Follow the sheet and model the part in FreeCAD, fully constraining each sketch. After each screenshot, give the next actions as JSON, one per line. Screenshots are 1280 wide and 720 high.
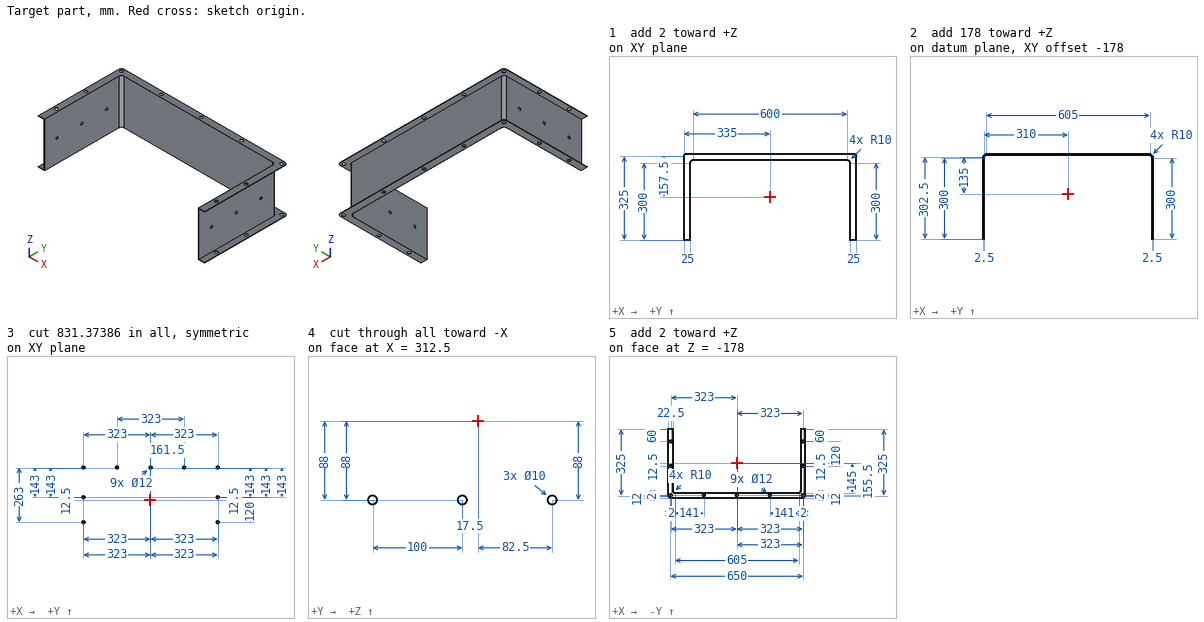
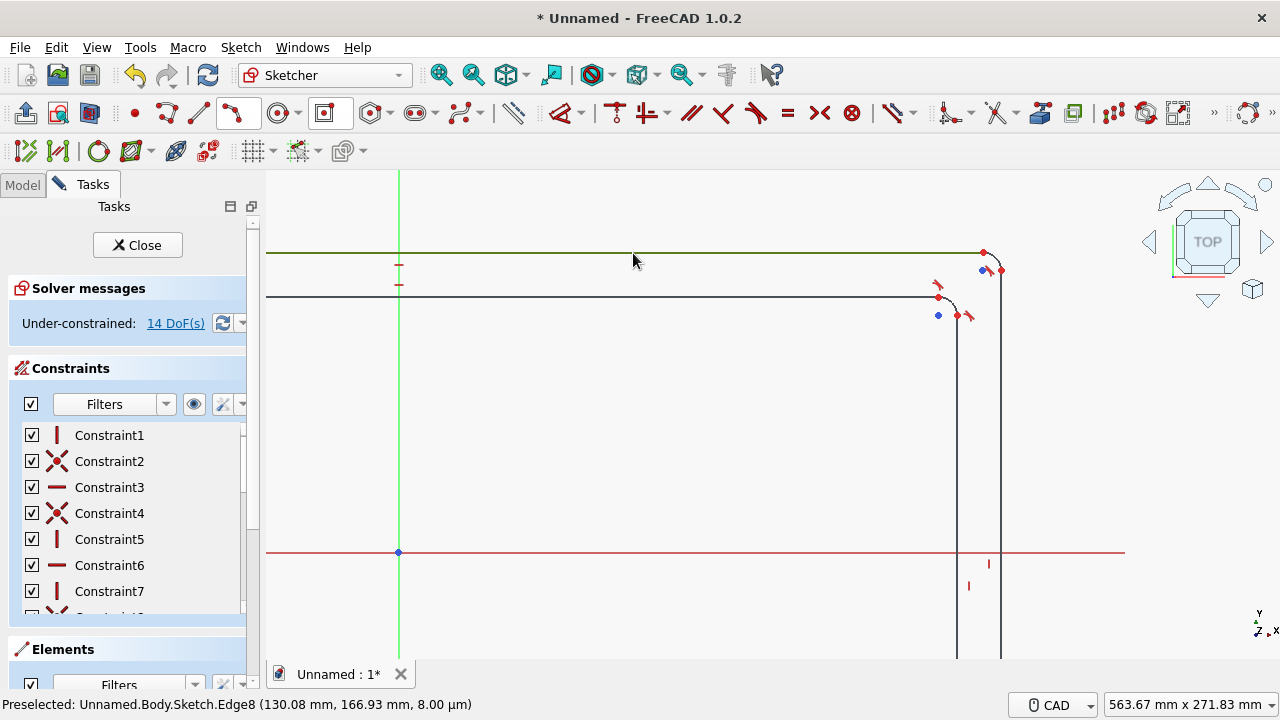
{"action": "left_click", "coordinate": [996, 258]}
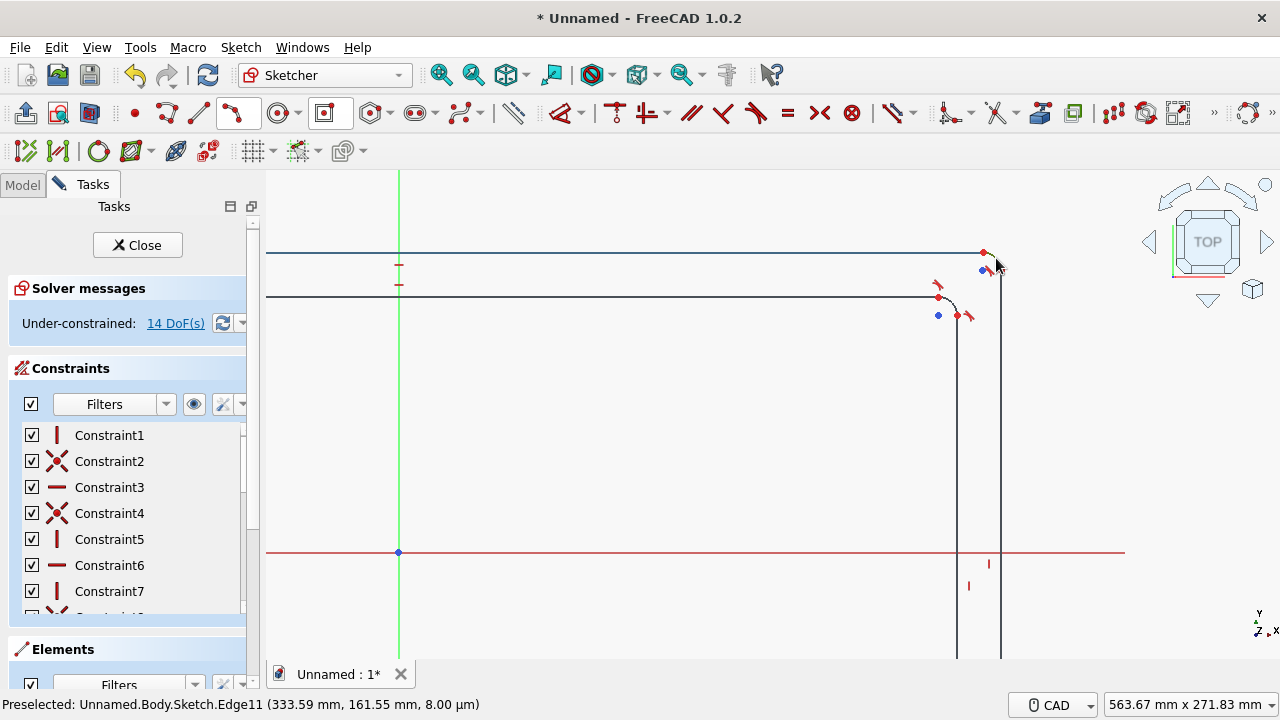
{"action": "key", "text": "t"}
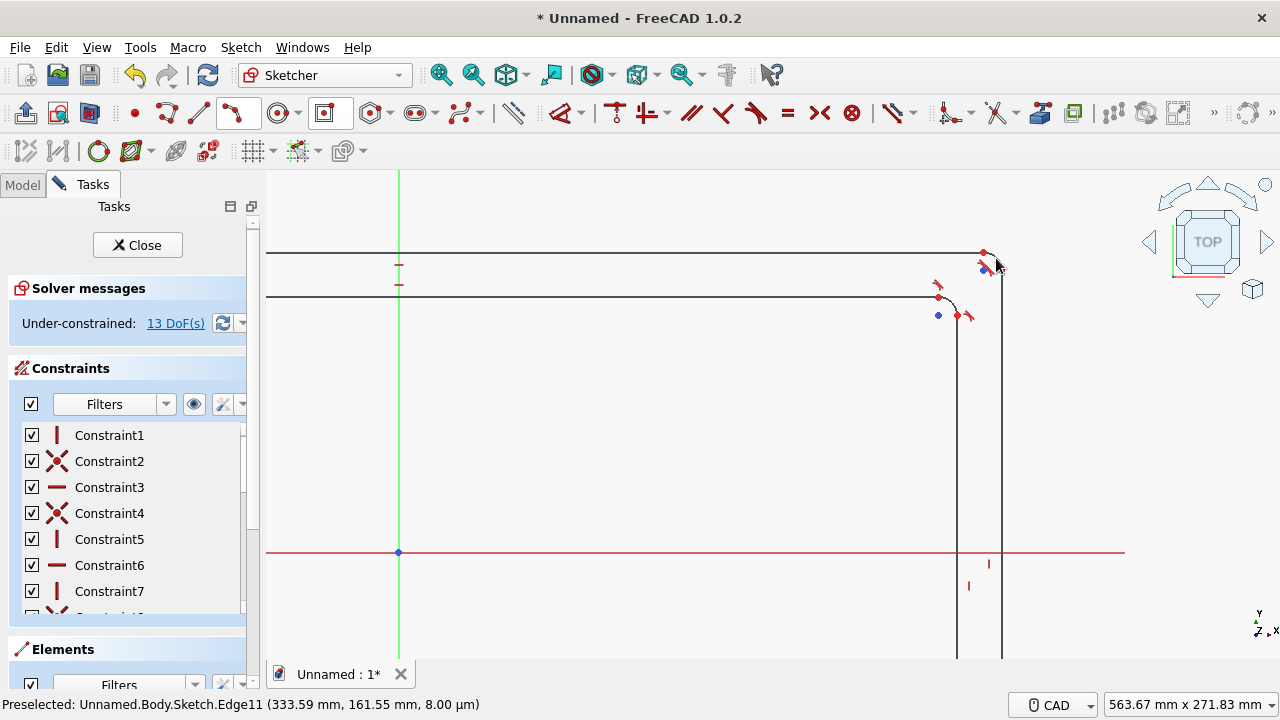
{"action": "left_click", "coordinate": [633, 253]}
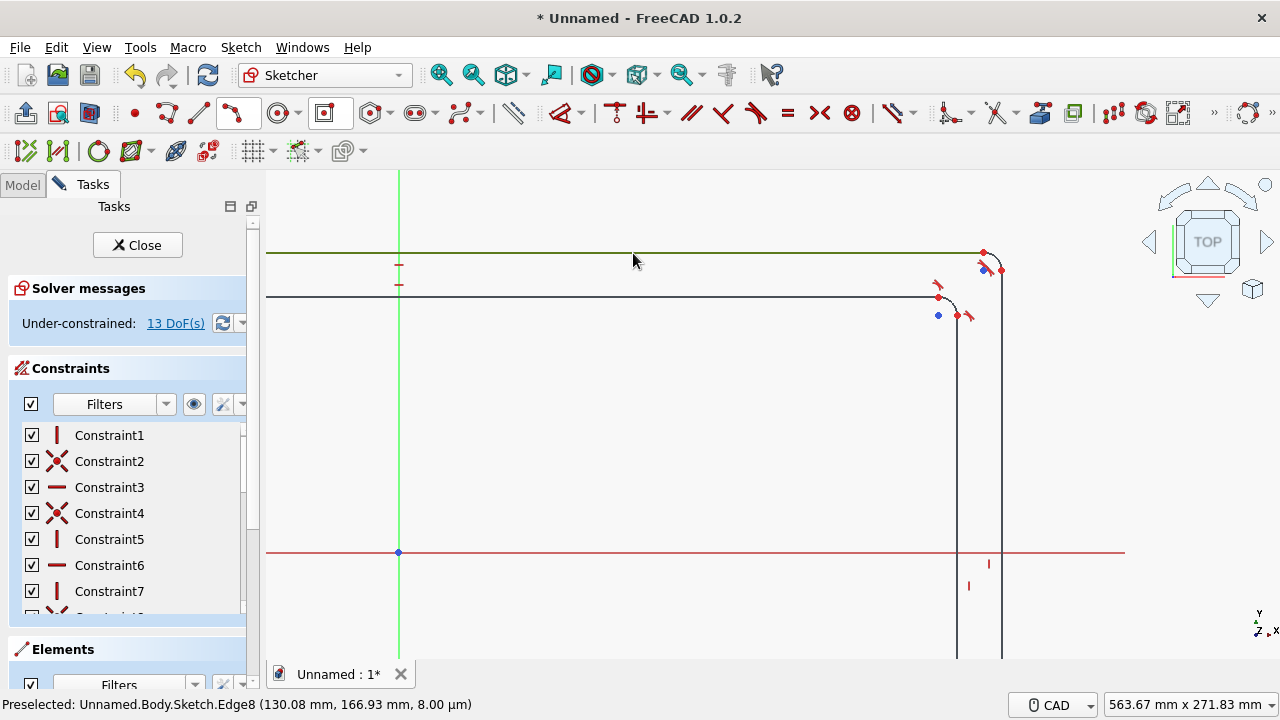
{"action": "scroll", "coordinate": [954, 302], "scroll_direction": "down", "scroll_amount": 4}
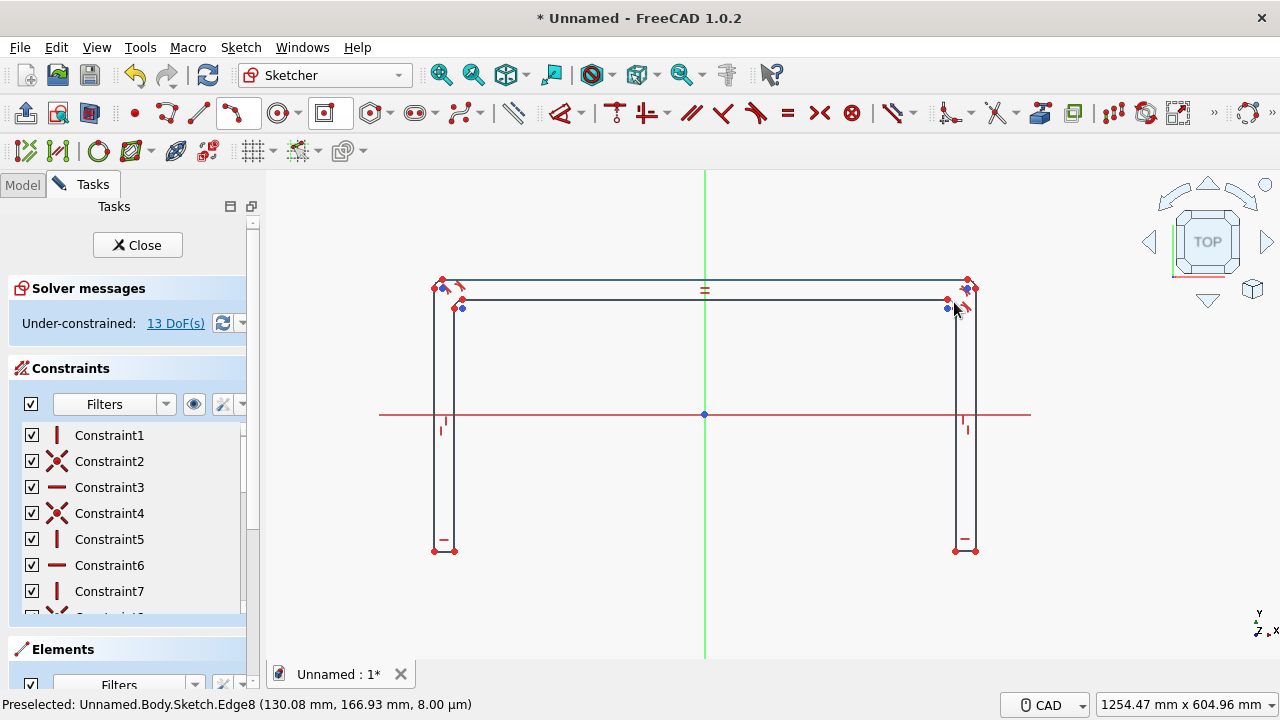
{"action": "scroll", "coordinate": [436, 282], "scroll_direction": "up", "scroll_amount": 4}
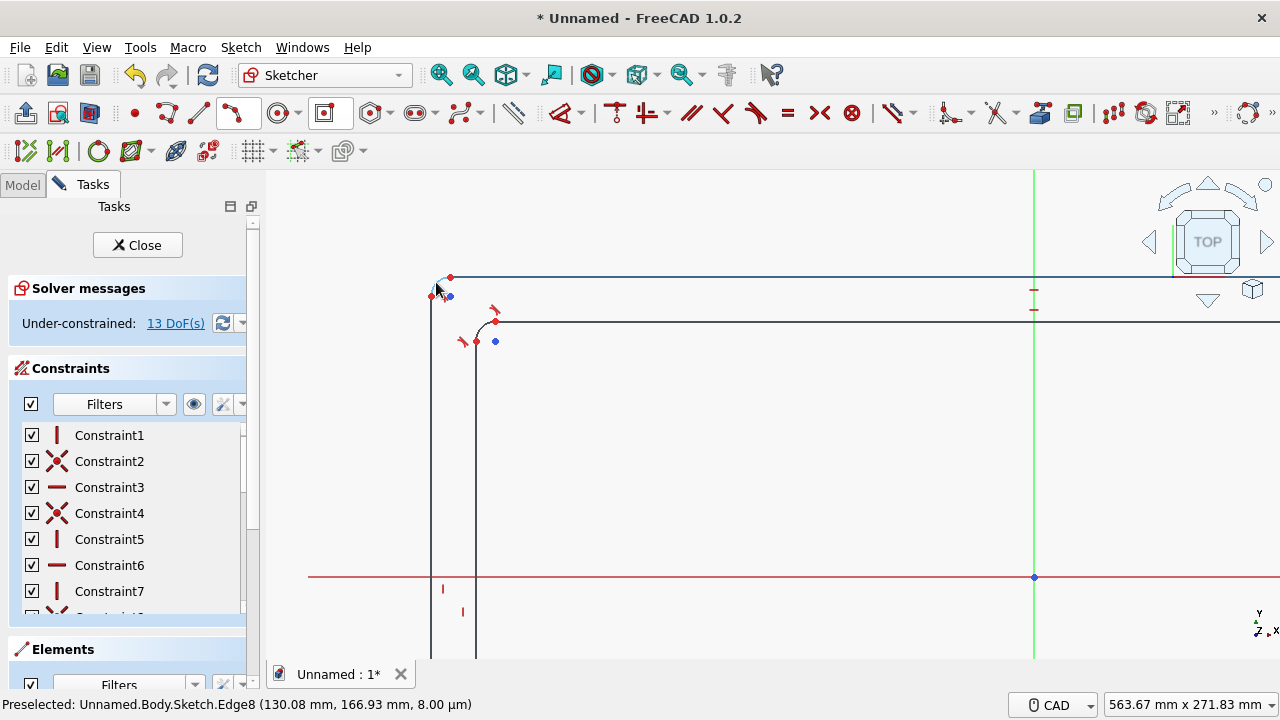
{"action": "left_click", "coordinate": [437, 283]}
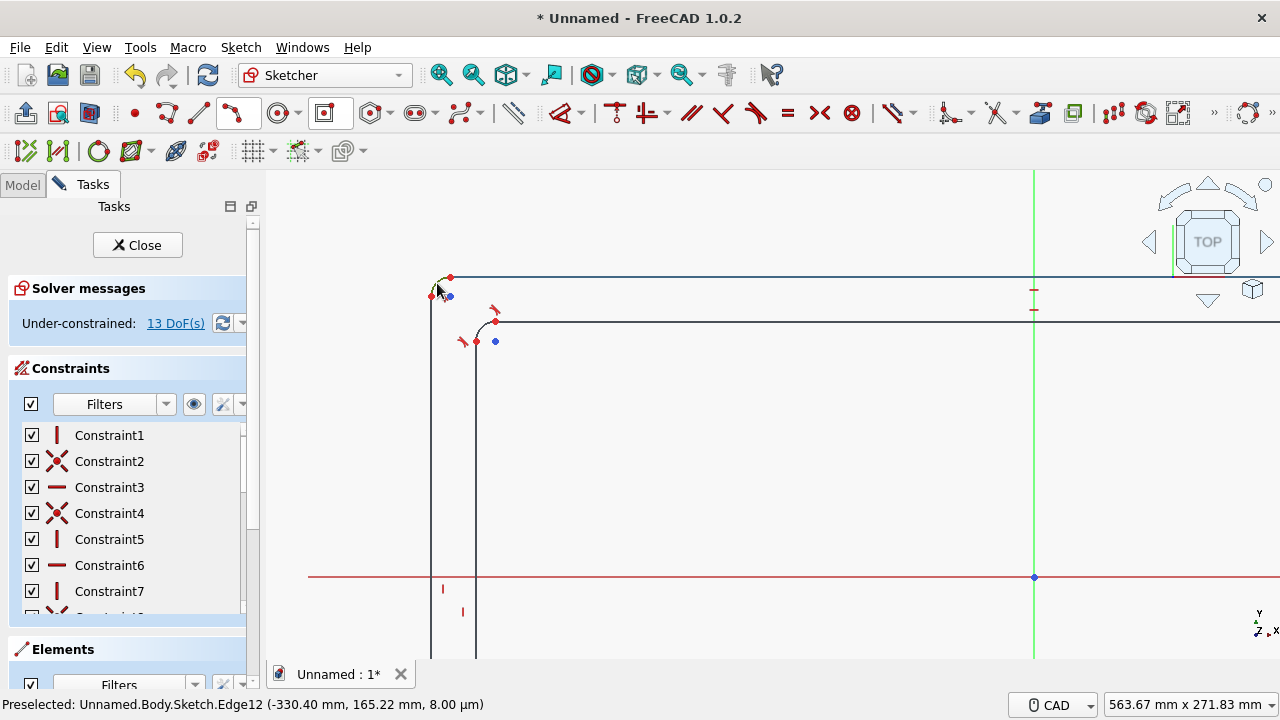
{"action": "left_click", "coordinate": [756, 114]}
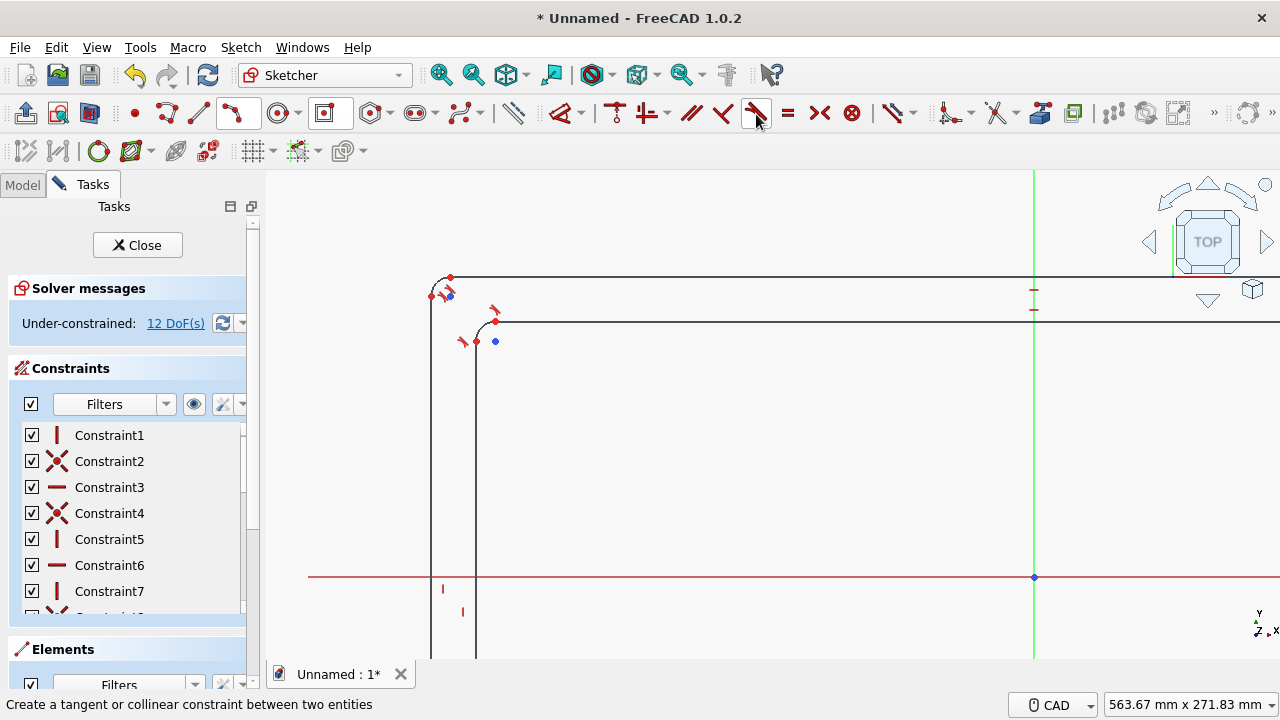
{"action": "scroll", "coordinate": [487, 324], "scroll_direction": "up", "scroll_amount": 3}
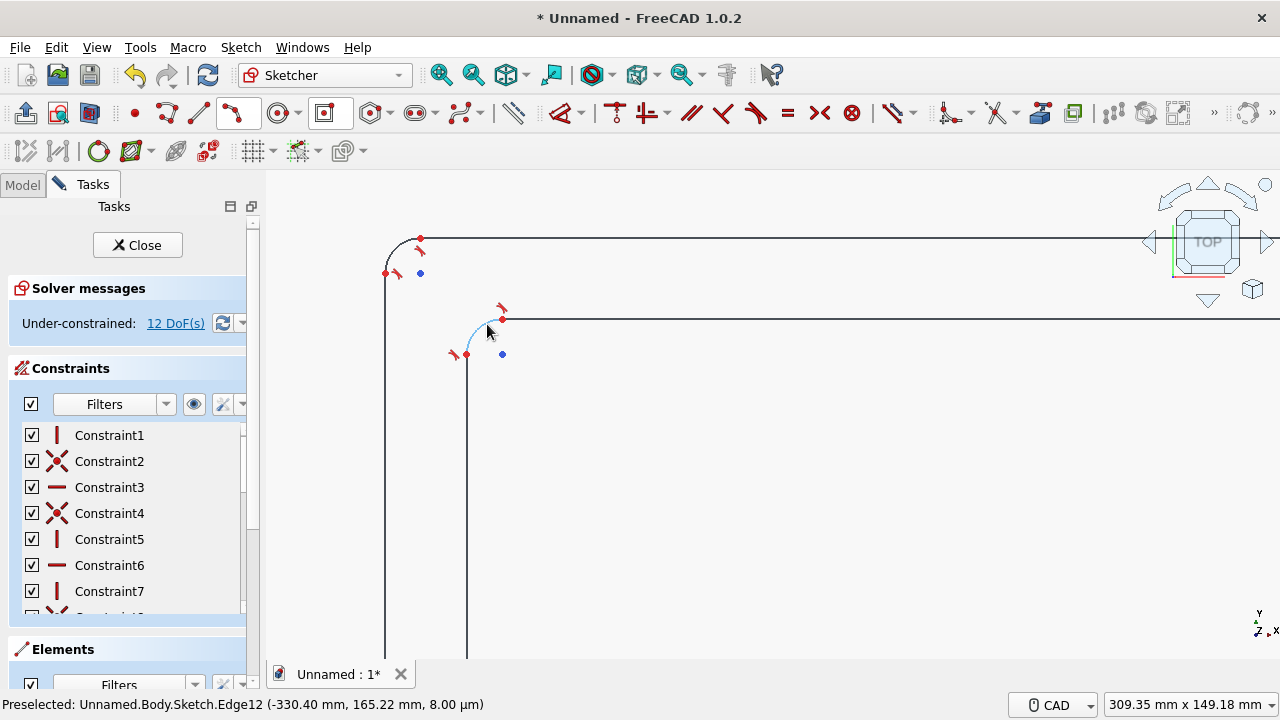
{"action": "left_click", "coordinate": [486, 323]}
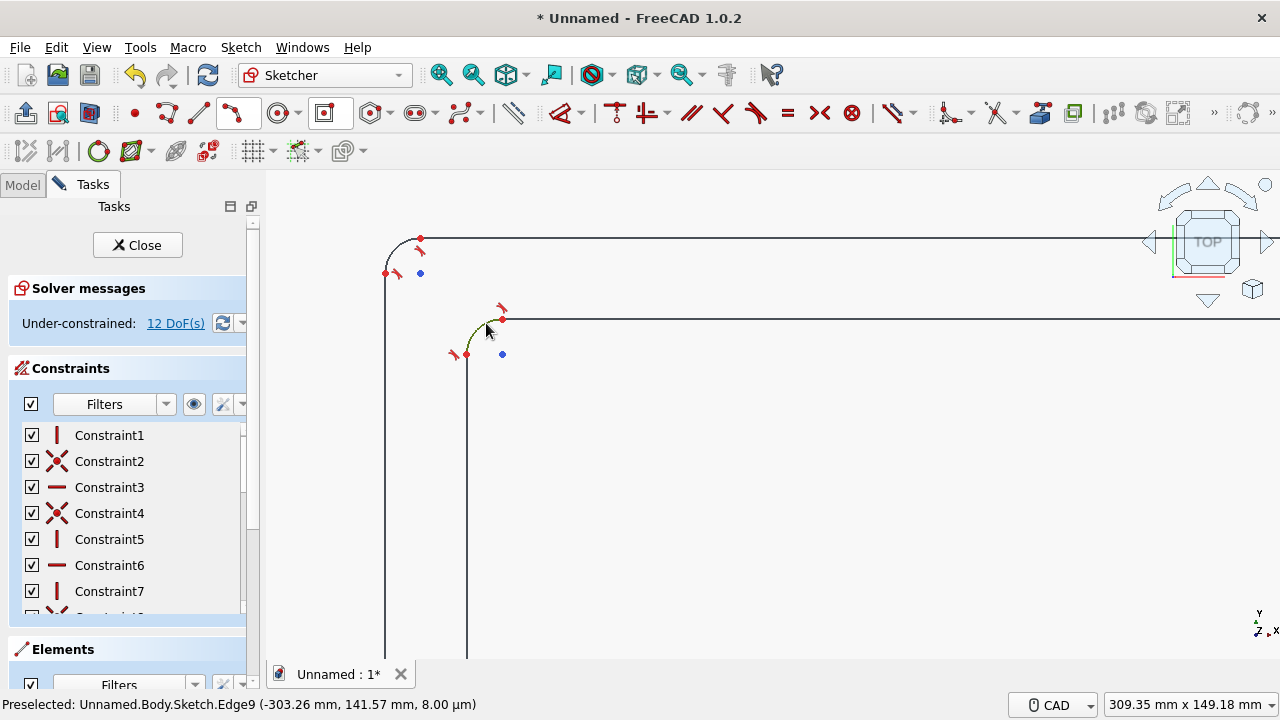
{"action": "scroll", "coordinate": [449, 293], "scroll_direction": "down", "scroll_amount": 7}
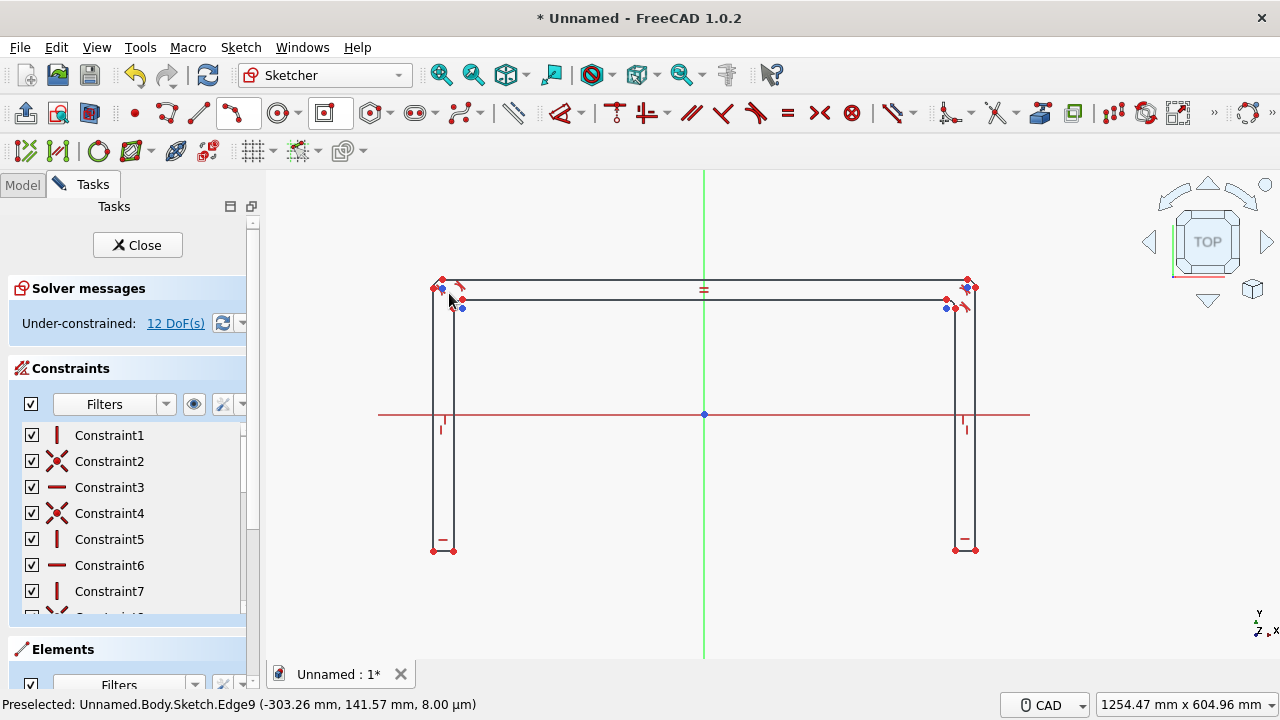
{"action": "scroll", "coordinate": [954, 304], "scroll_direction": "up", "scroll_amount": 7}